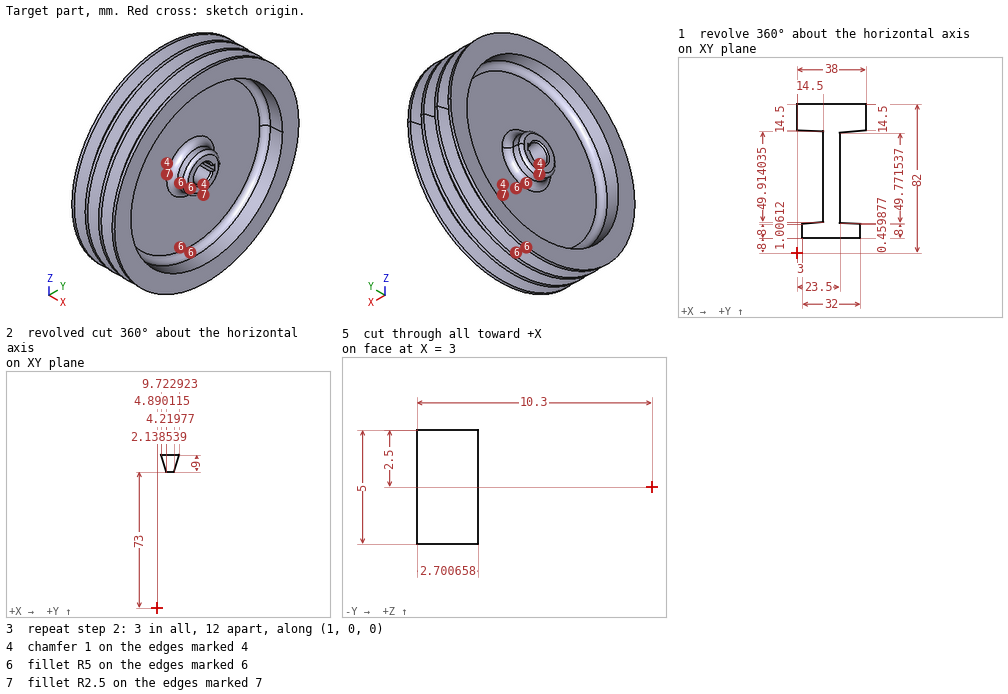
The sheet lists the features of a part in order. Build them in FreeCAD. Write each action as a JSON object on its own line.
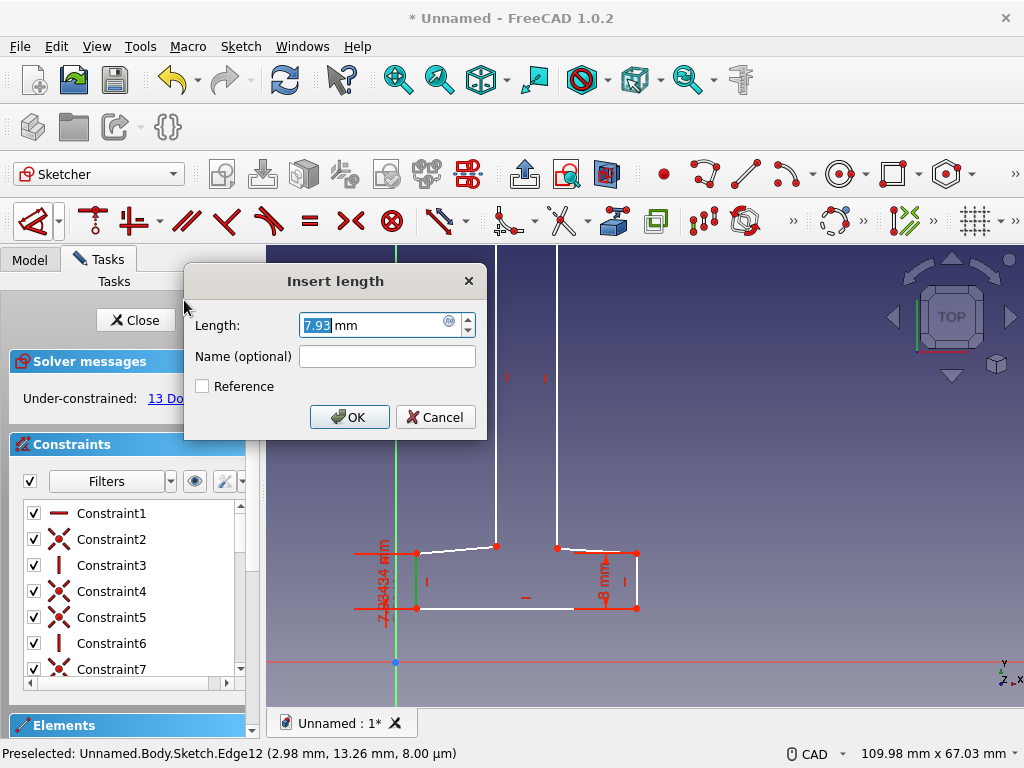
{"action": "type", "text": "8"}
{"action": "key", "text": "Return"}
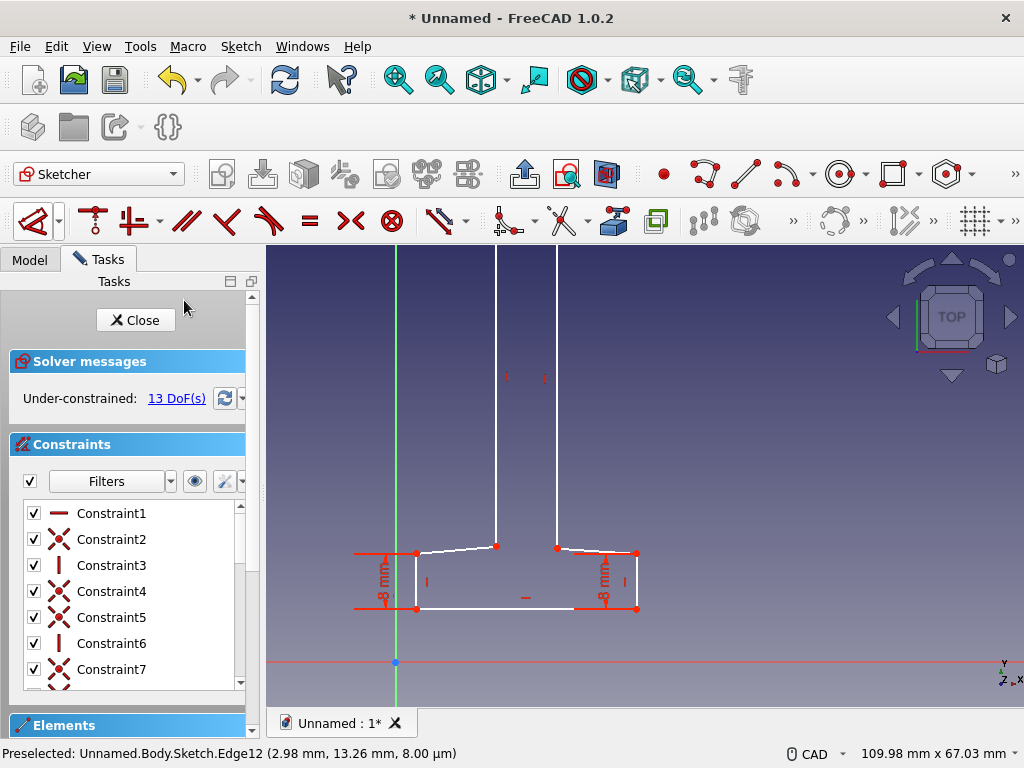
{"action": "left_click", "coordinate": [482, 609]}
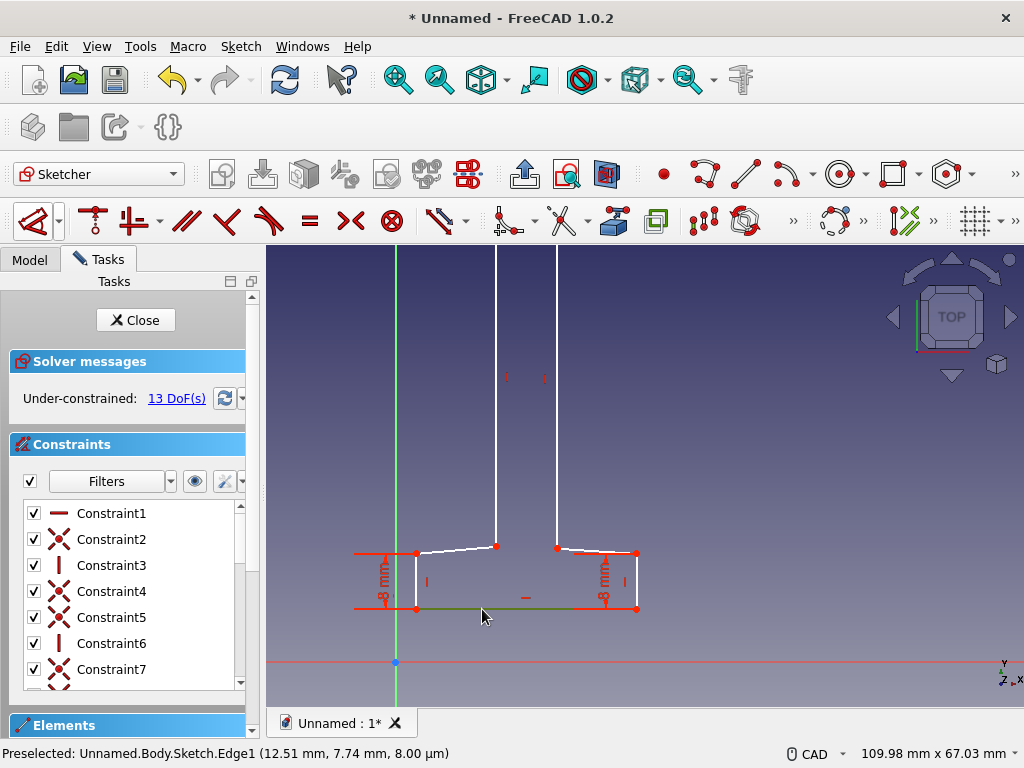
{"action": "key", "text": "l"}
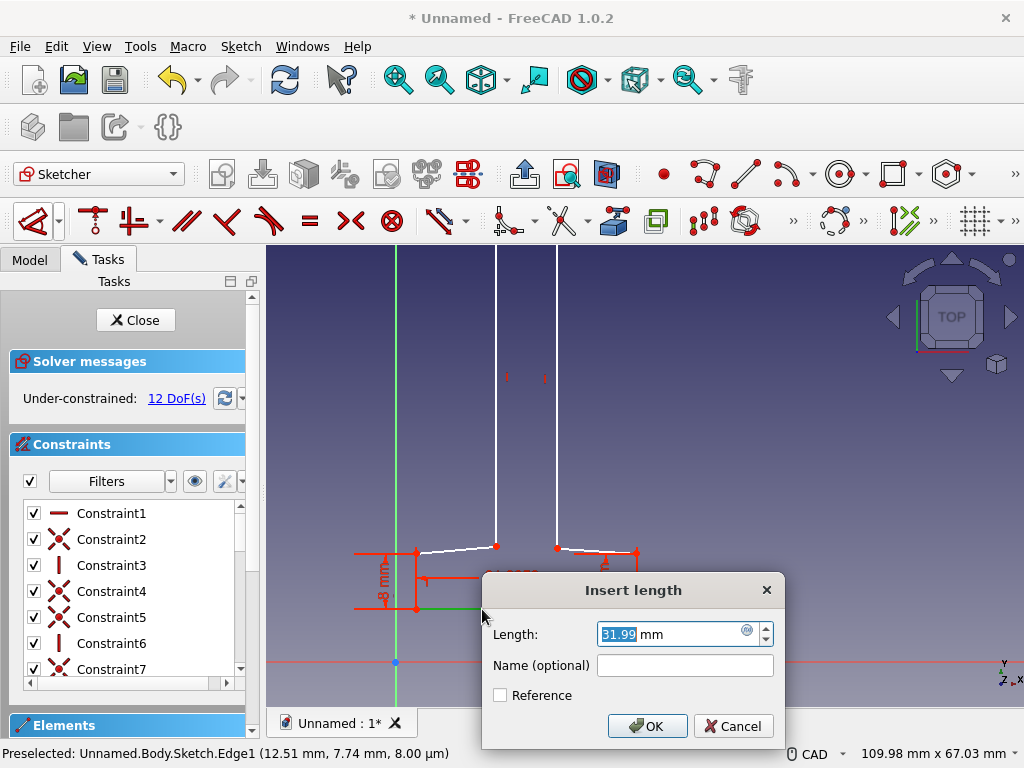
{"action": "type", "text": "32"}
{"action": "key", "text": "Return"}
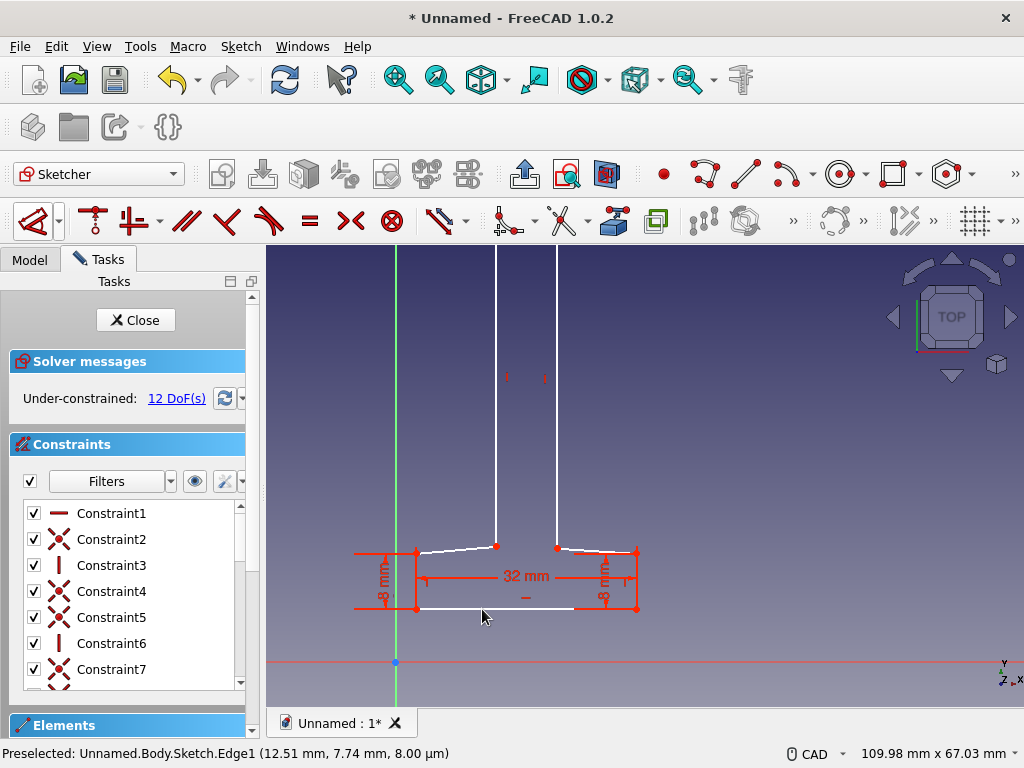
{"action": "scroll", "coordinate": [637, 593], "scroll_direction": "down", "scroll_amount": 3}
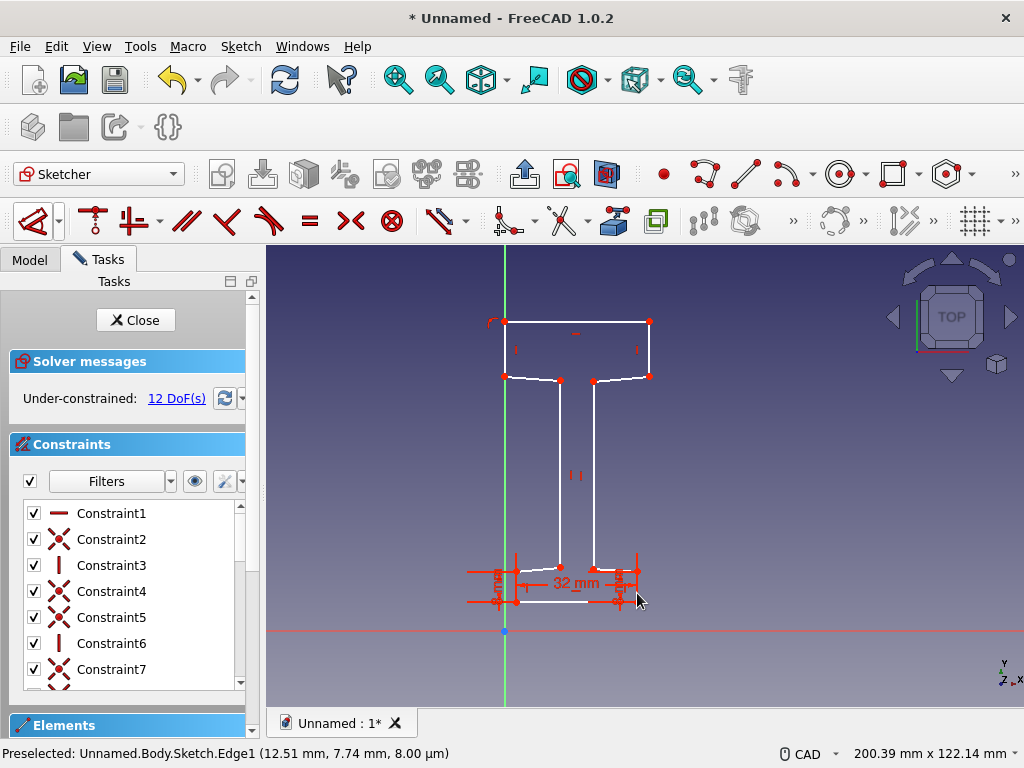
{"action": "left_click", "coordinate": [606, 322]}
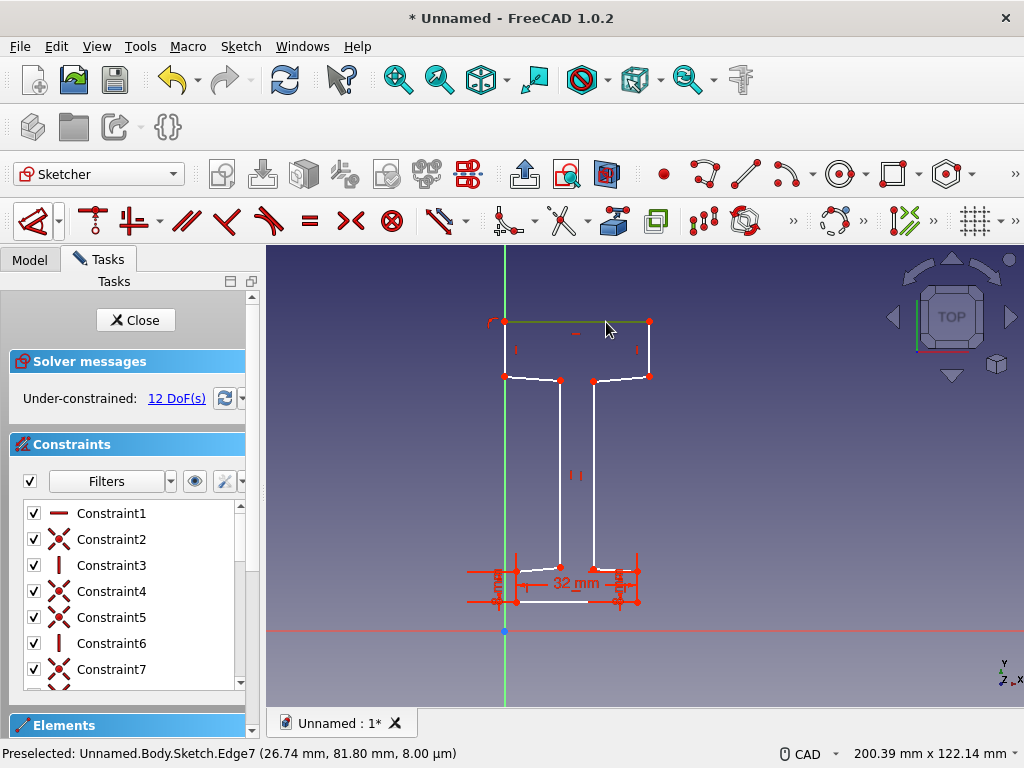
{"action": "left_click", "coordinate": [58, 222]}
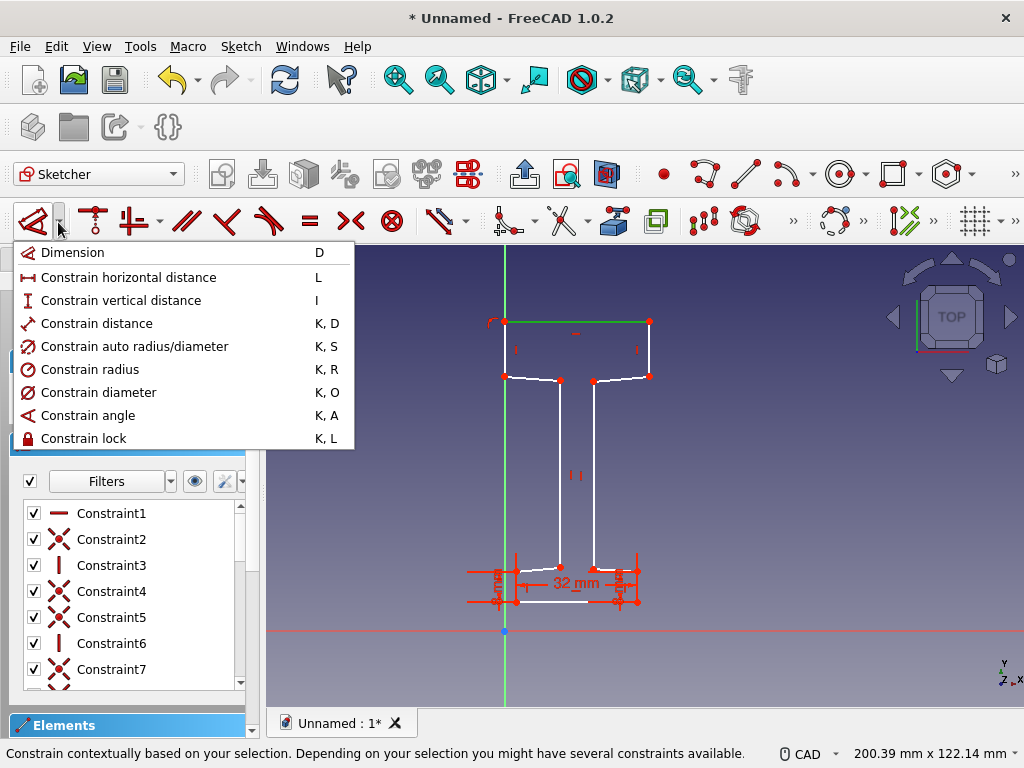
{"action": "left_click", "coordinate": [184, 278]}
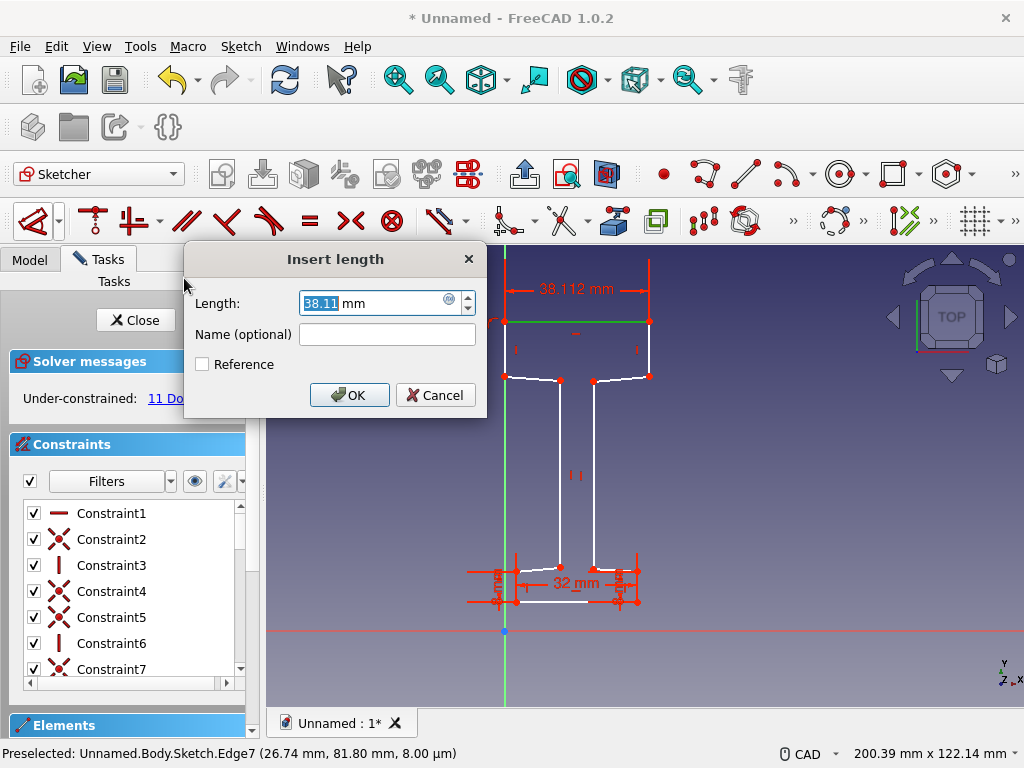
{"action": "type", "text": "38"}
{"action": "key", "text": "Return"}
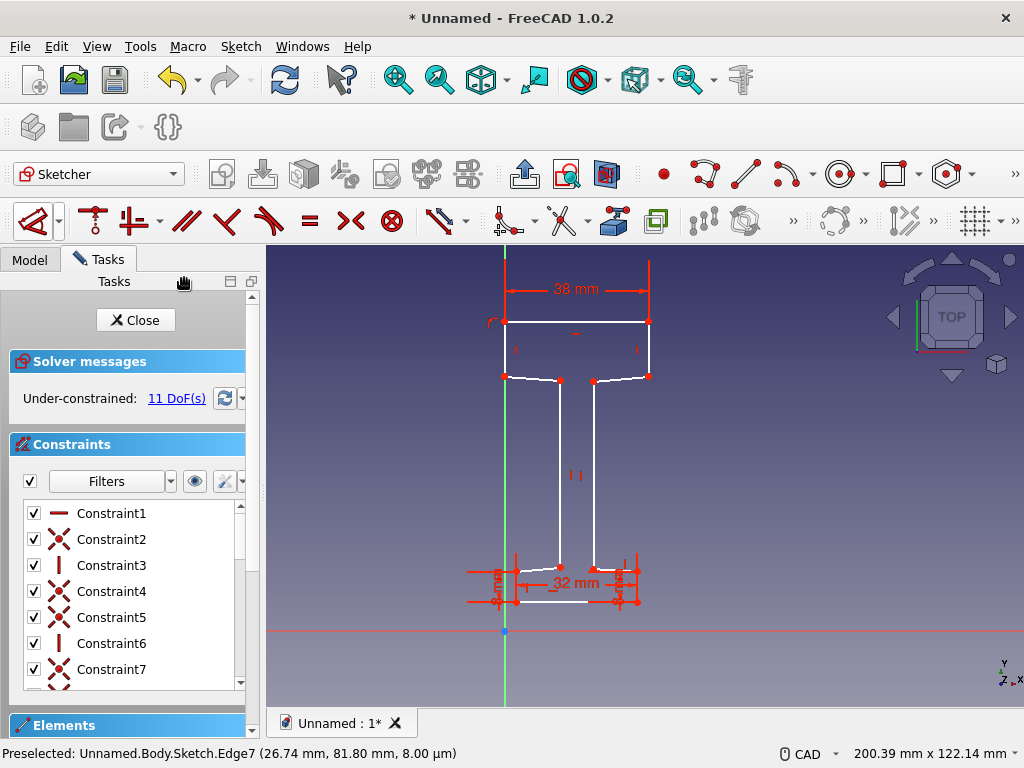
{"action": "scroll", "coordinate": [516, 602], "scroll_direction": "up", "scroll_amount": 7}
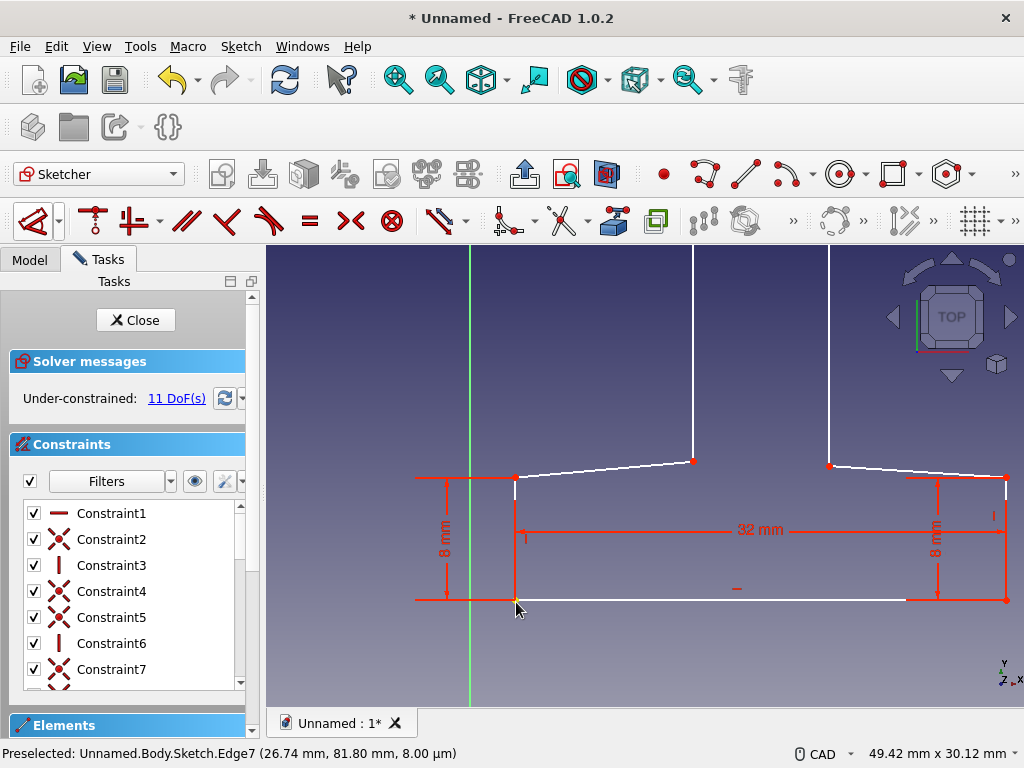
{"action": "left_click", "coordinate": [515, 600]}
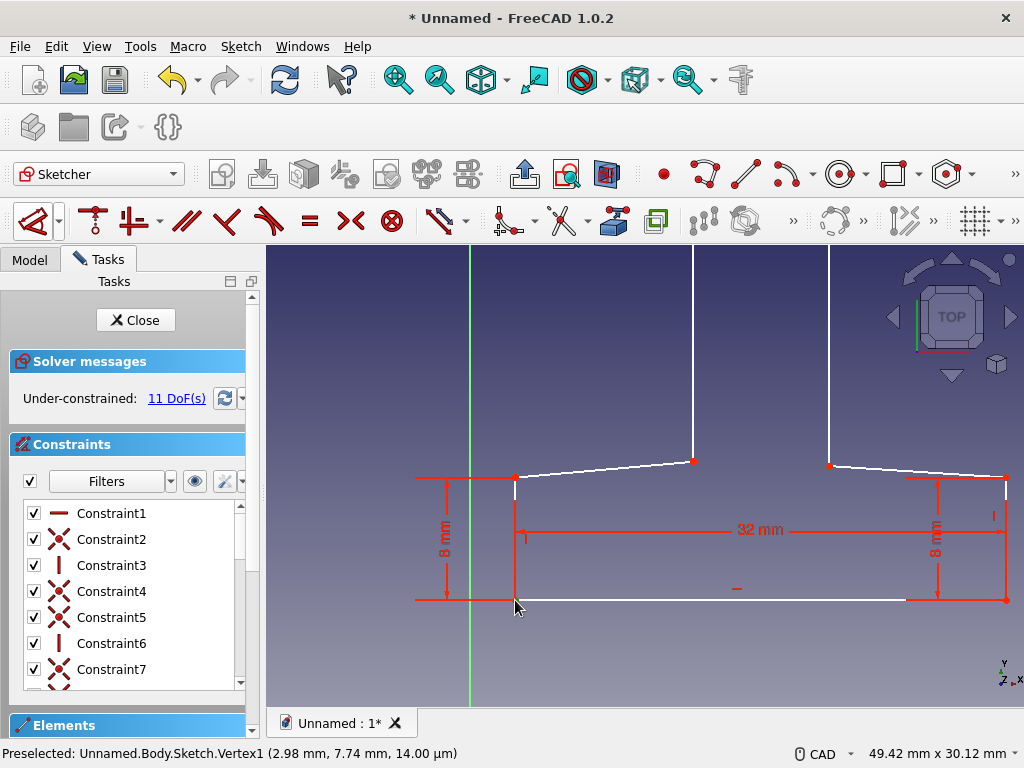
{"action": "key", "text": "l"}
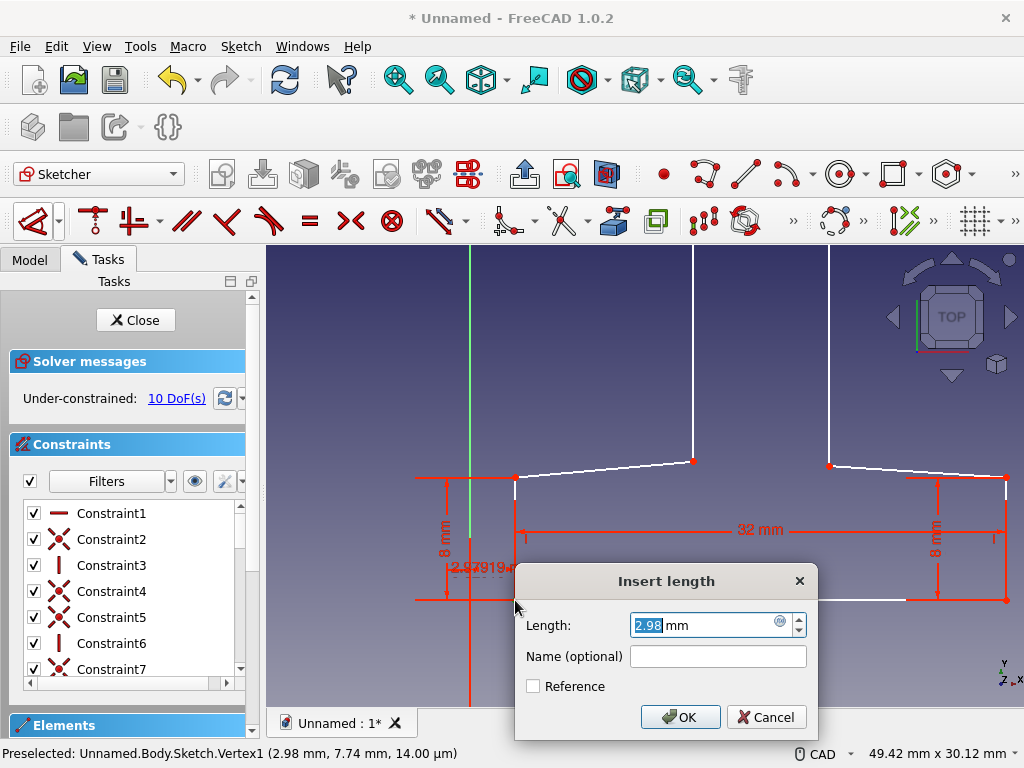
{"action": "type", "text": "3"}
{"action": "key", "text": "Return"}